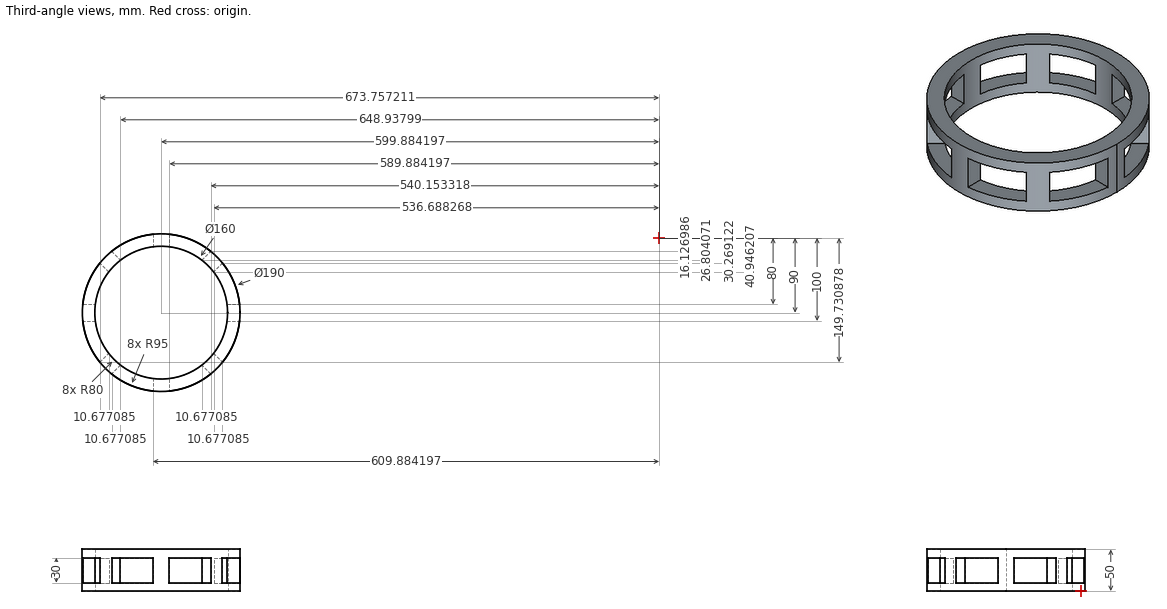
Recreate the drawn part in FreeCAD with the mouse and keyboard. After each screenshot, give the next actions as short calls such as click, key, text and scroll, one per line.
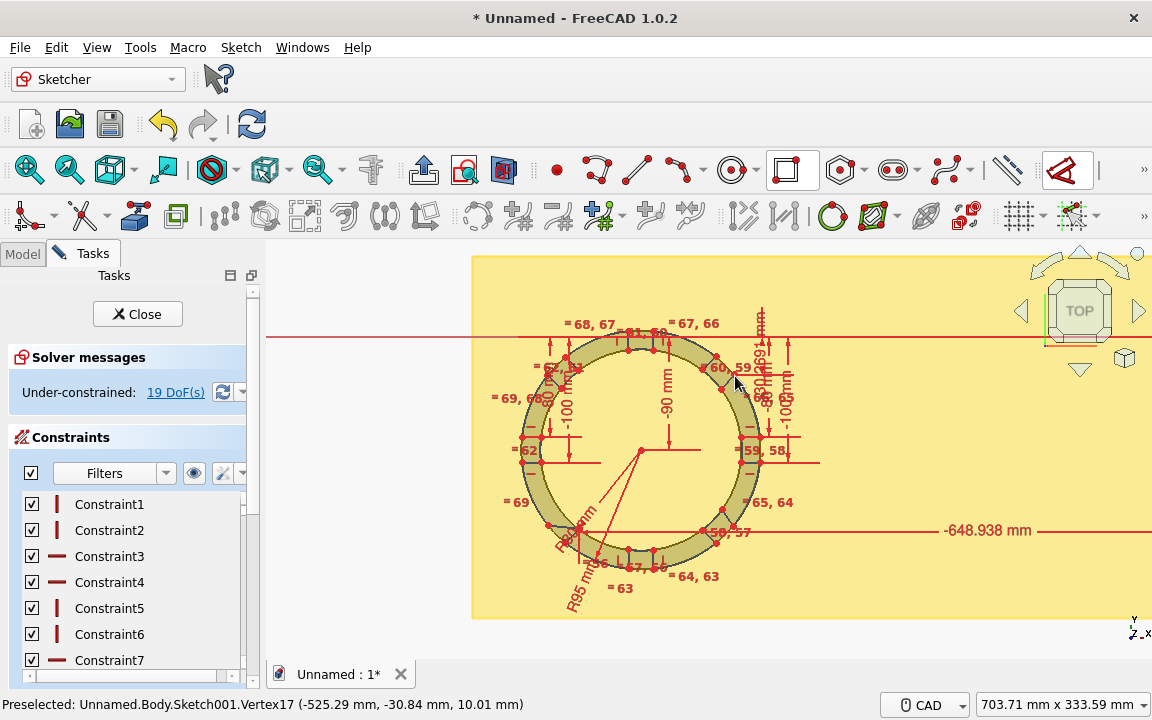
click(722, 390)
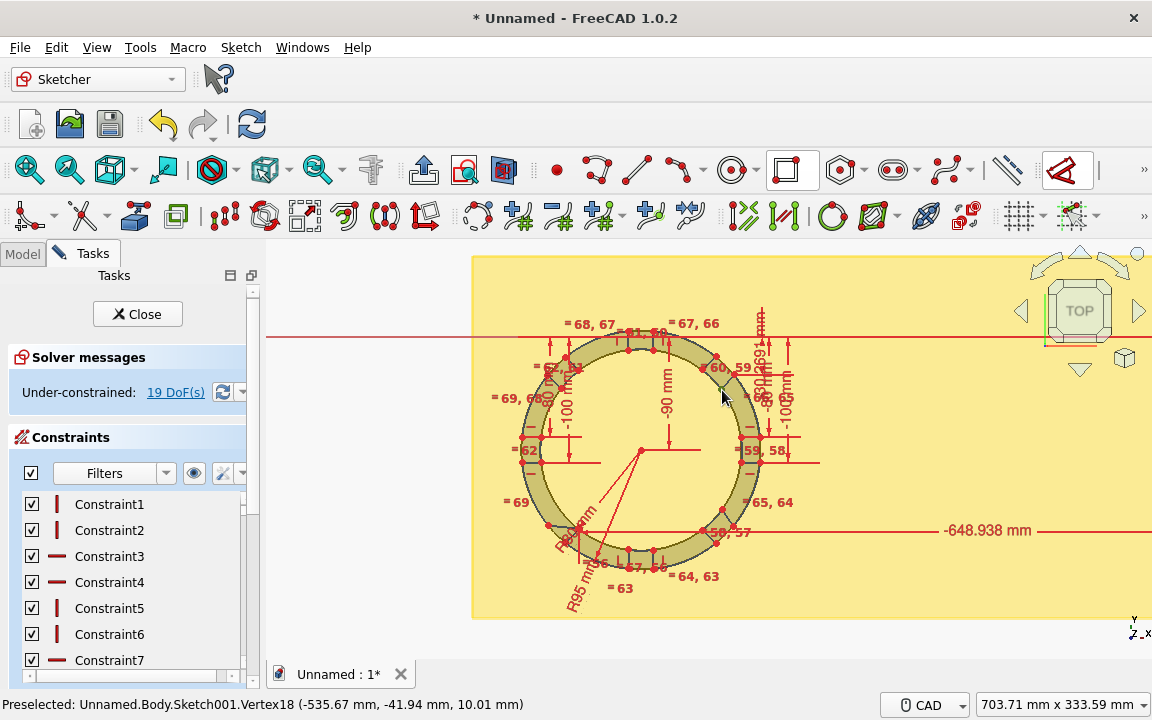
key(i)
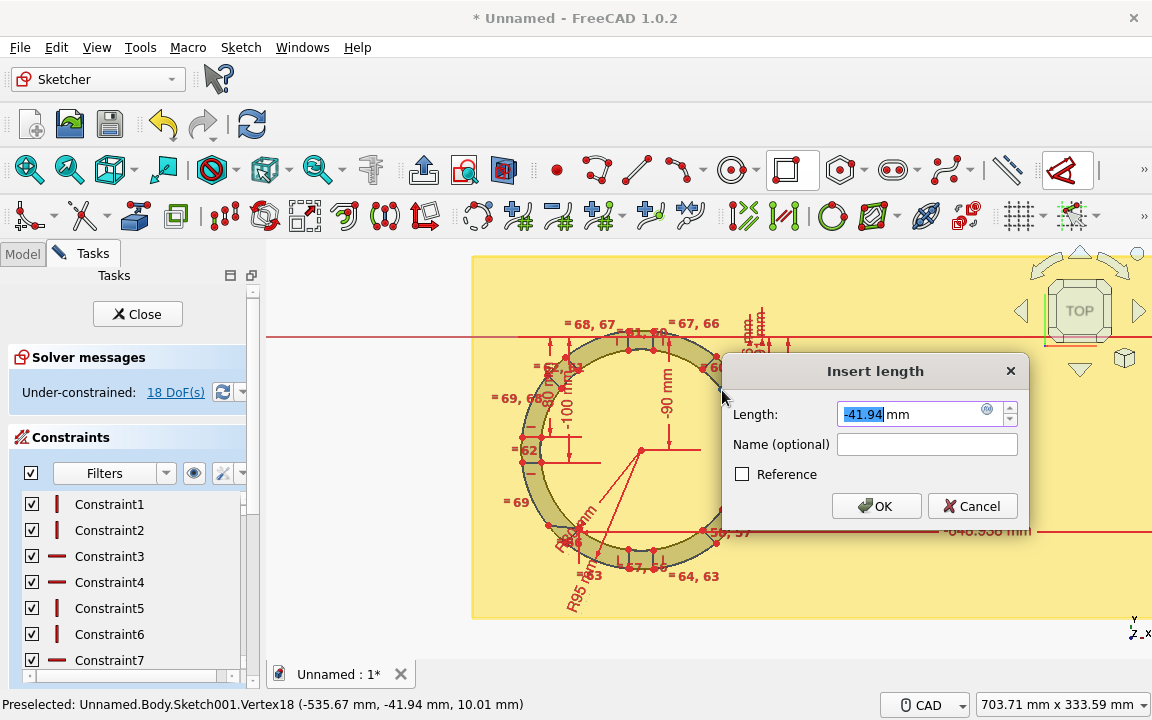
text(-40.946207)
key(Return)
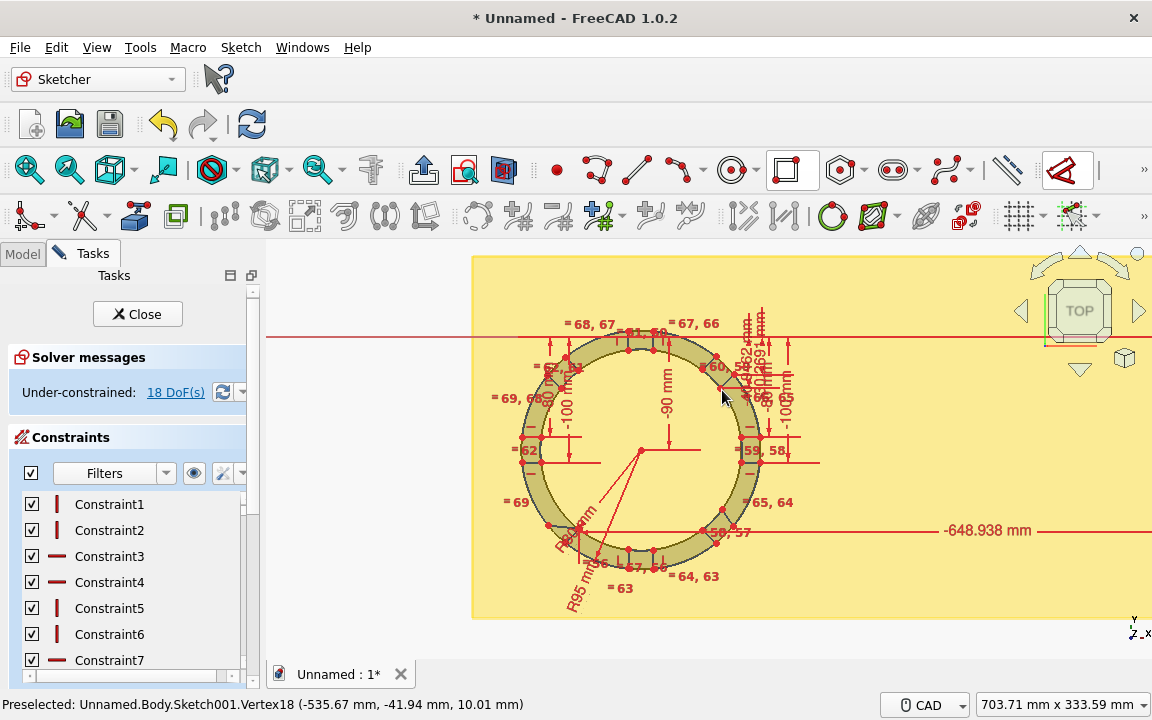
click(702, 370)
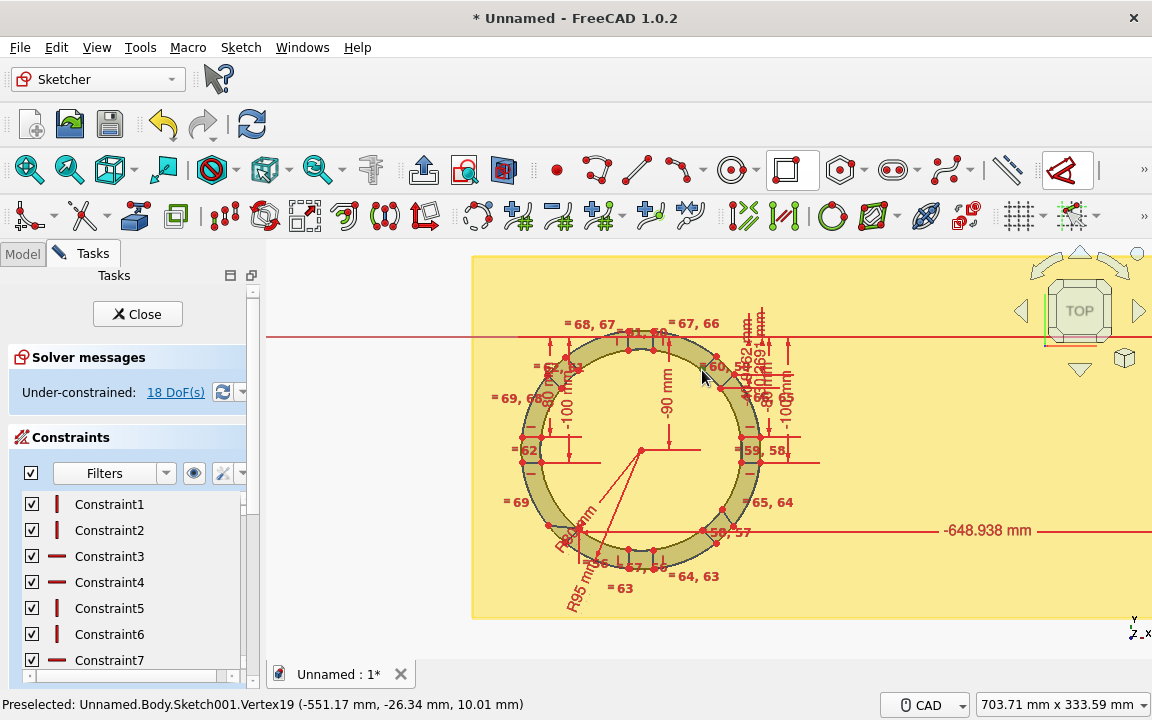
click(1088, 170)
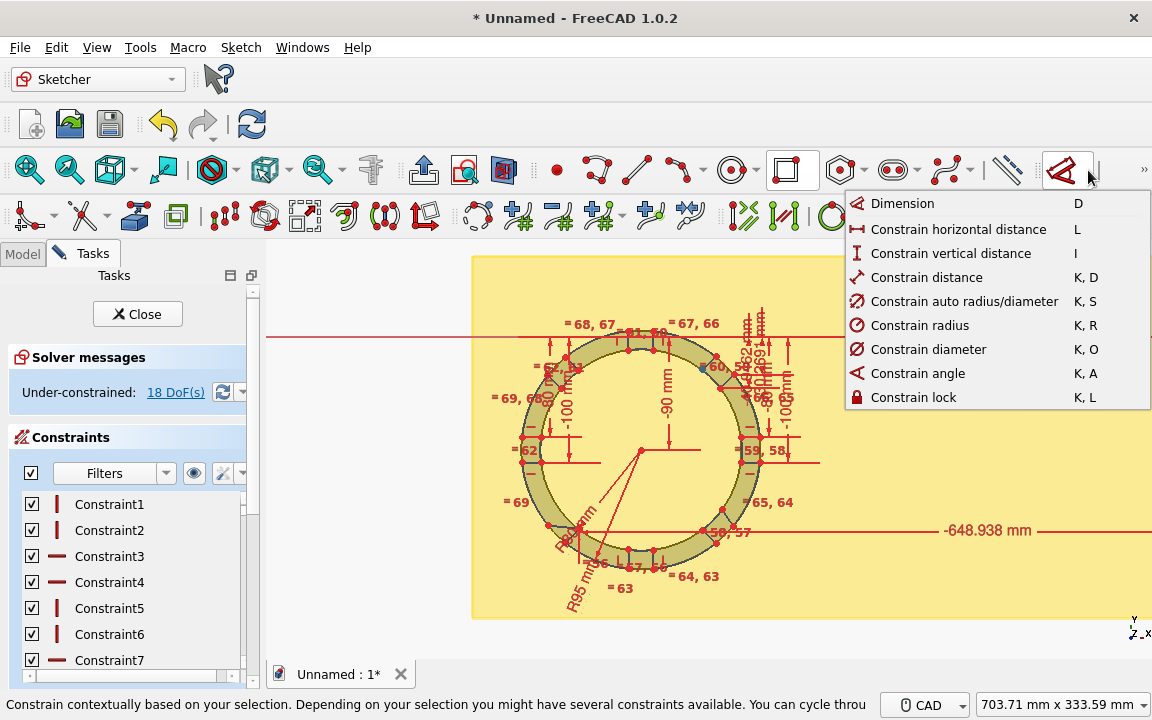
click(998, 253)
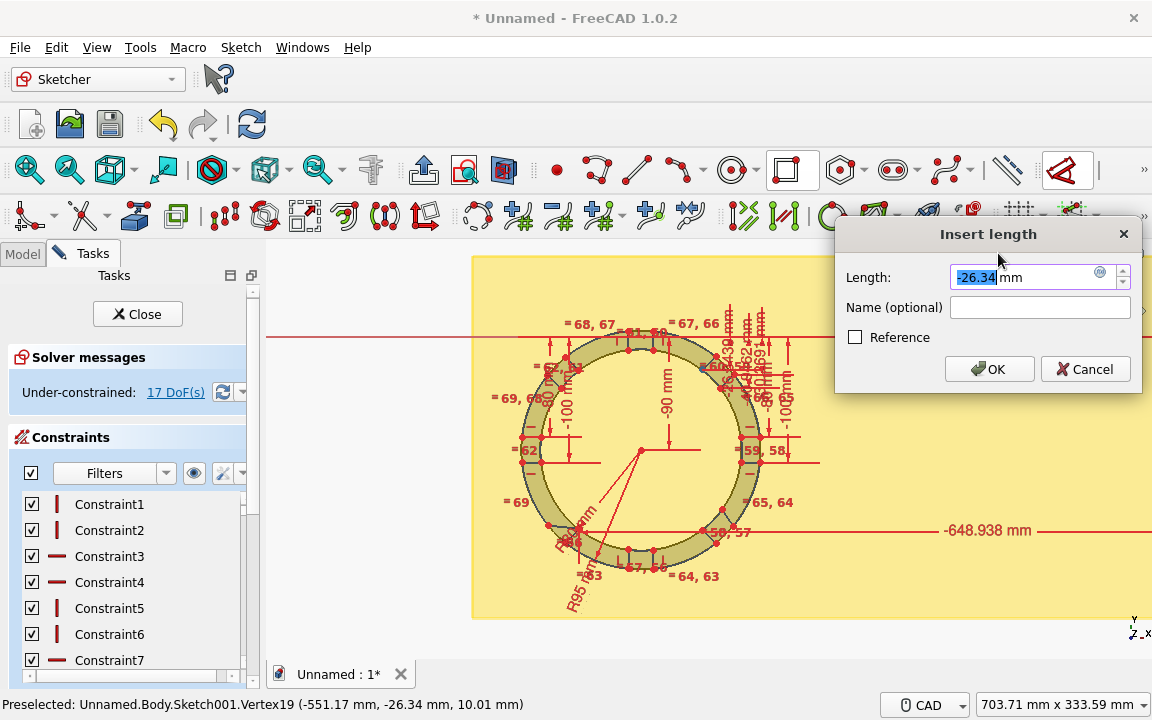
text(-26.804071)
key(Return)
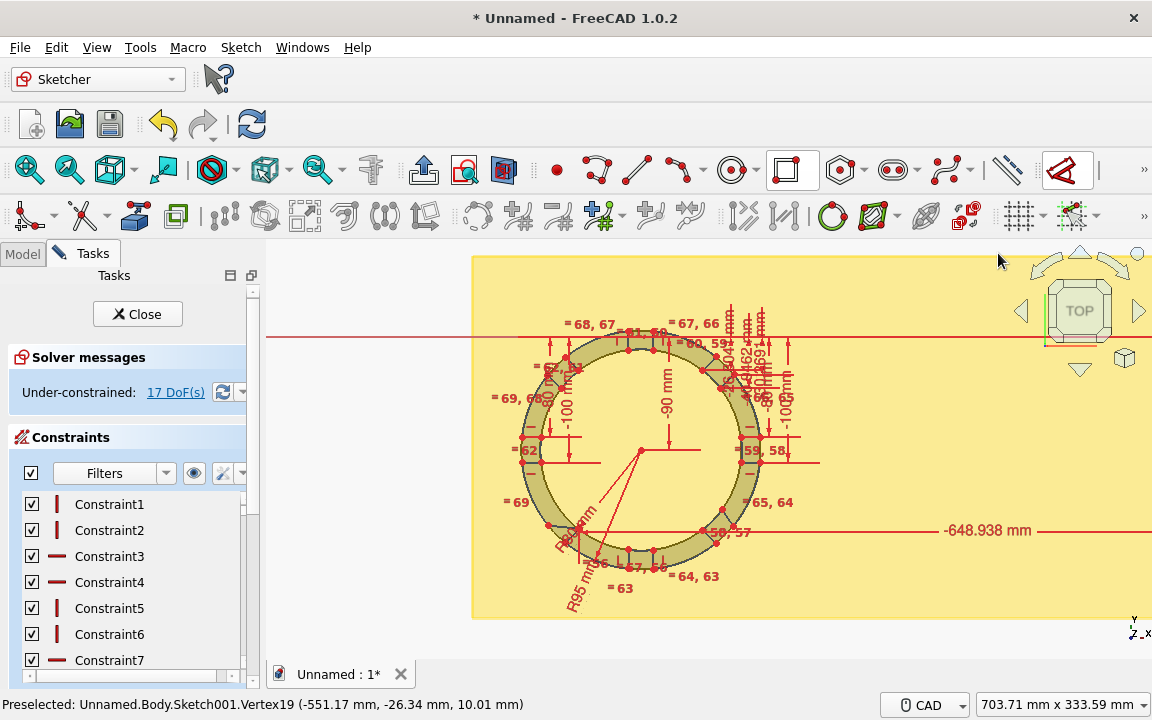
scroll(716, 357, up, 4)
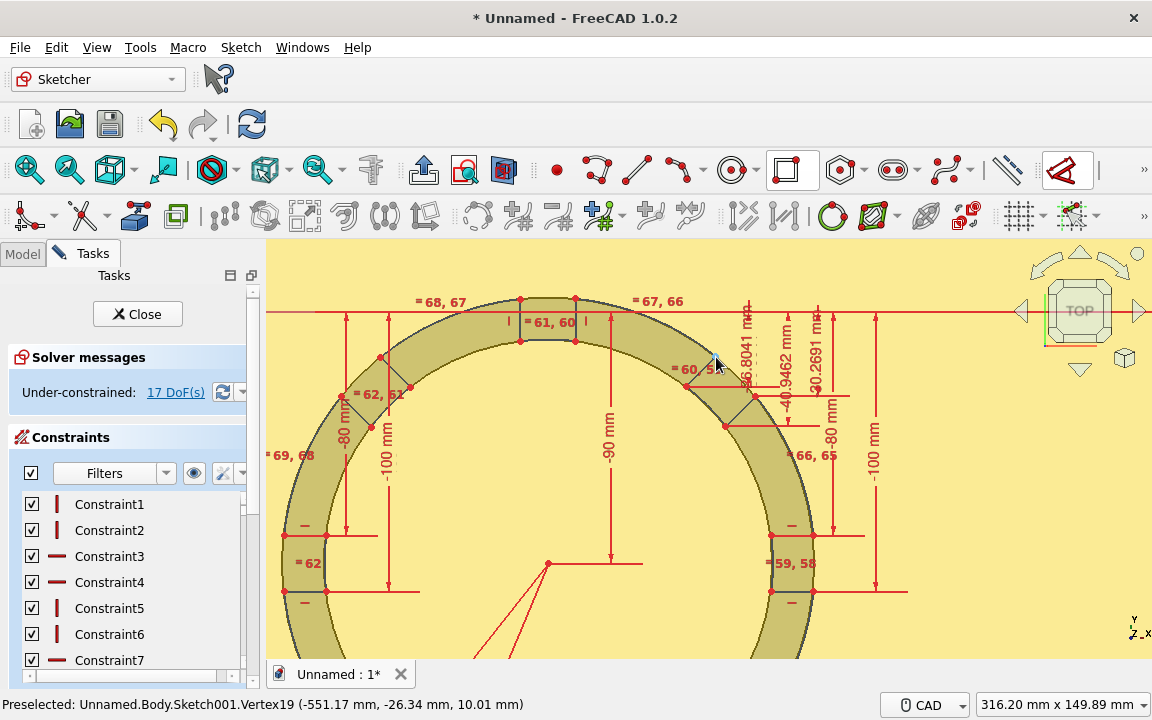
click(716, 356)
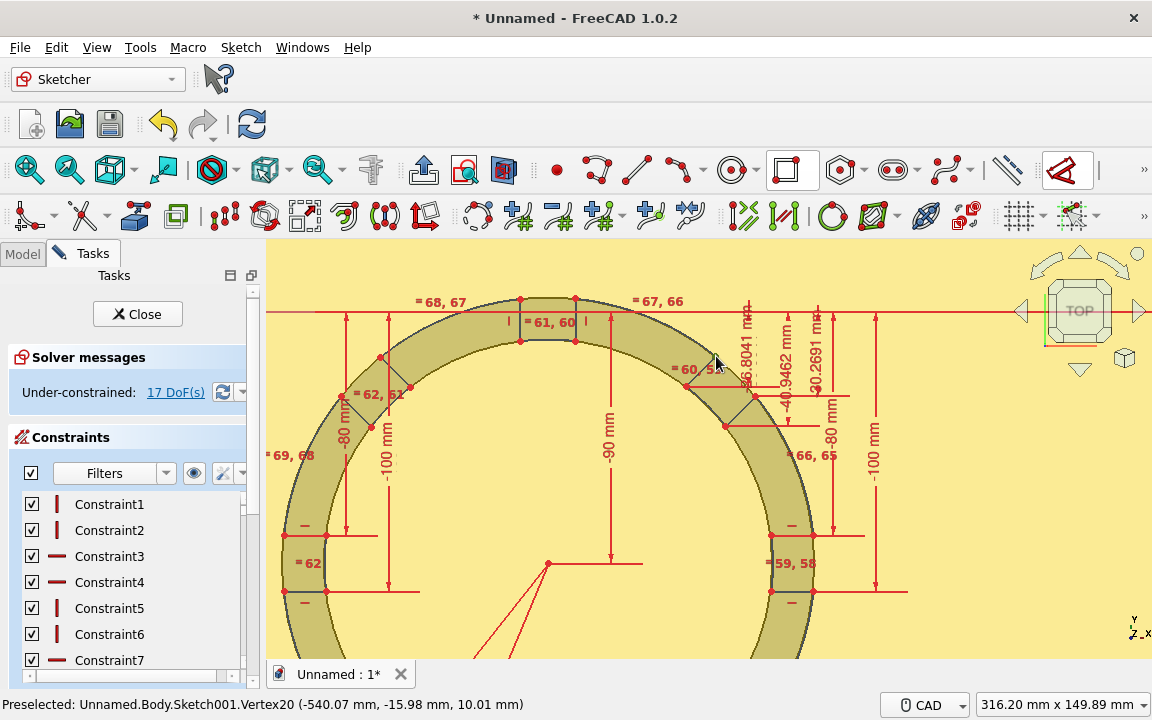
key(i)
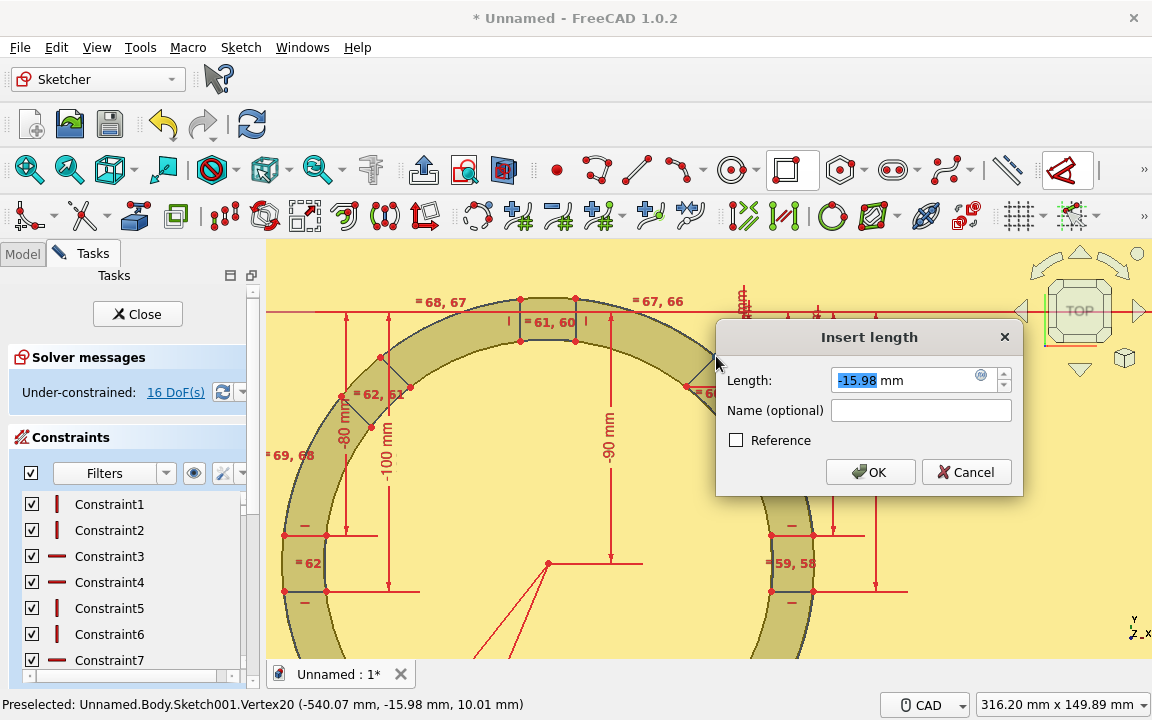
text(-16.126986)
key(Return)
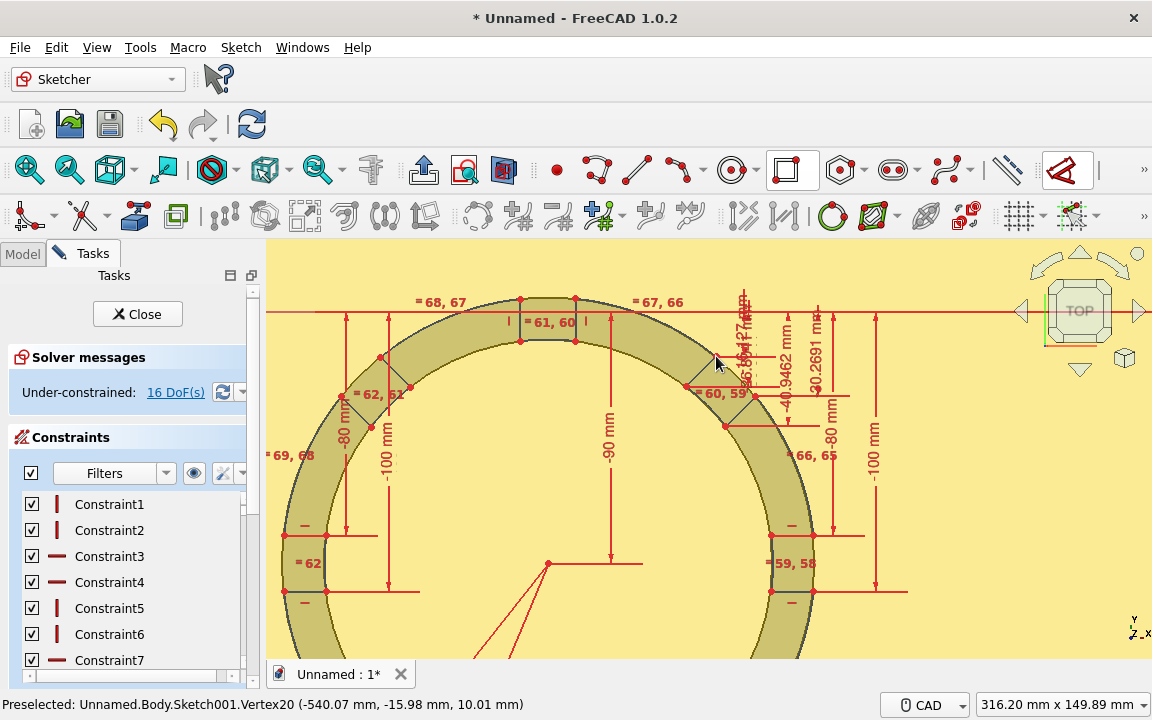
click(381, 357)